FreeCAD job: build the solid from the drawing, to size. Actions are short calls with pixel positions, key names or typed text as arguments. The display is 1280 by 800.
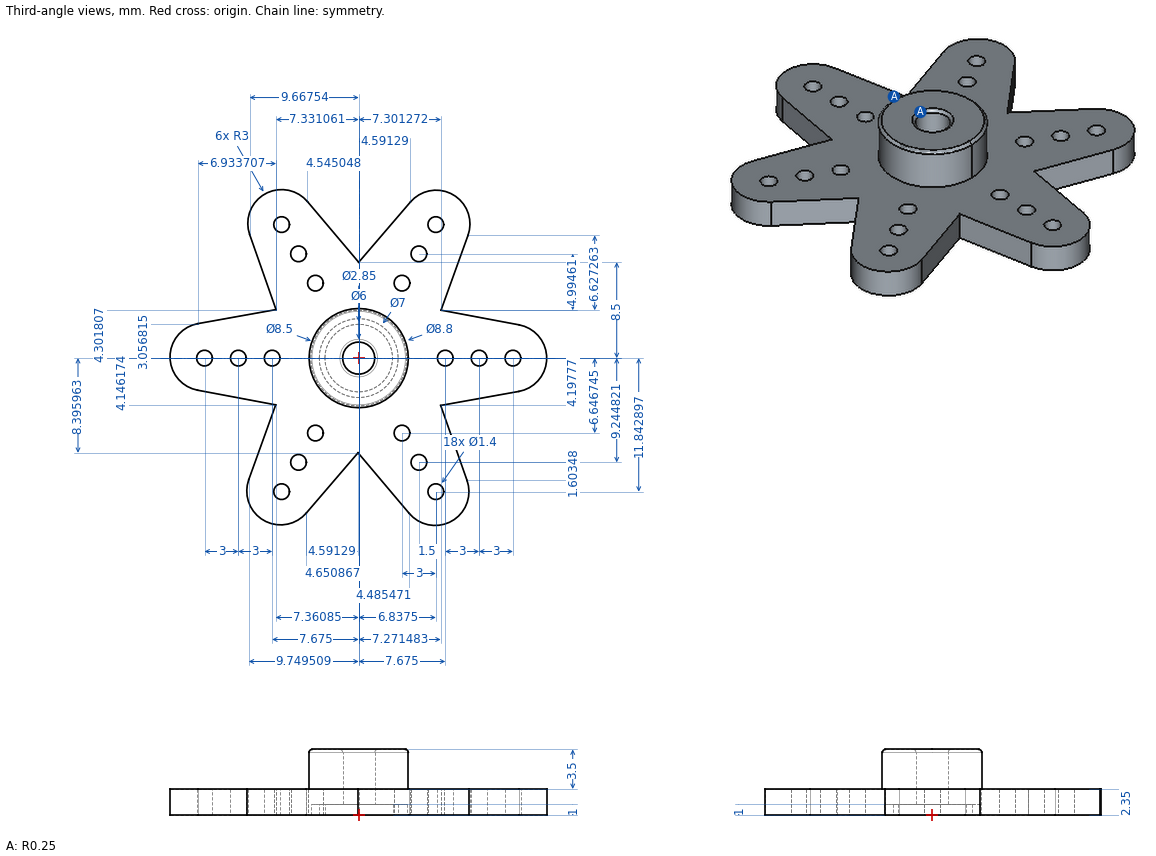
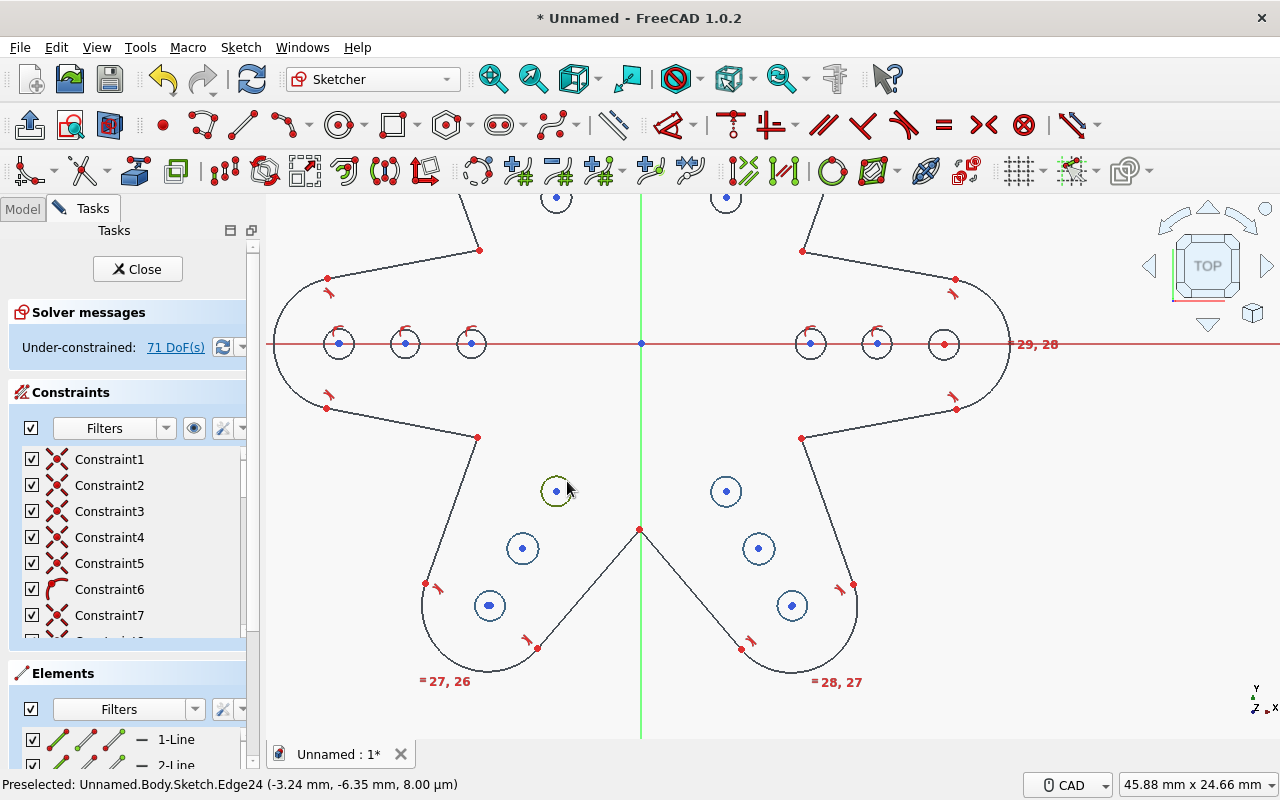
scroll(955, 334, up, 2)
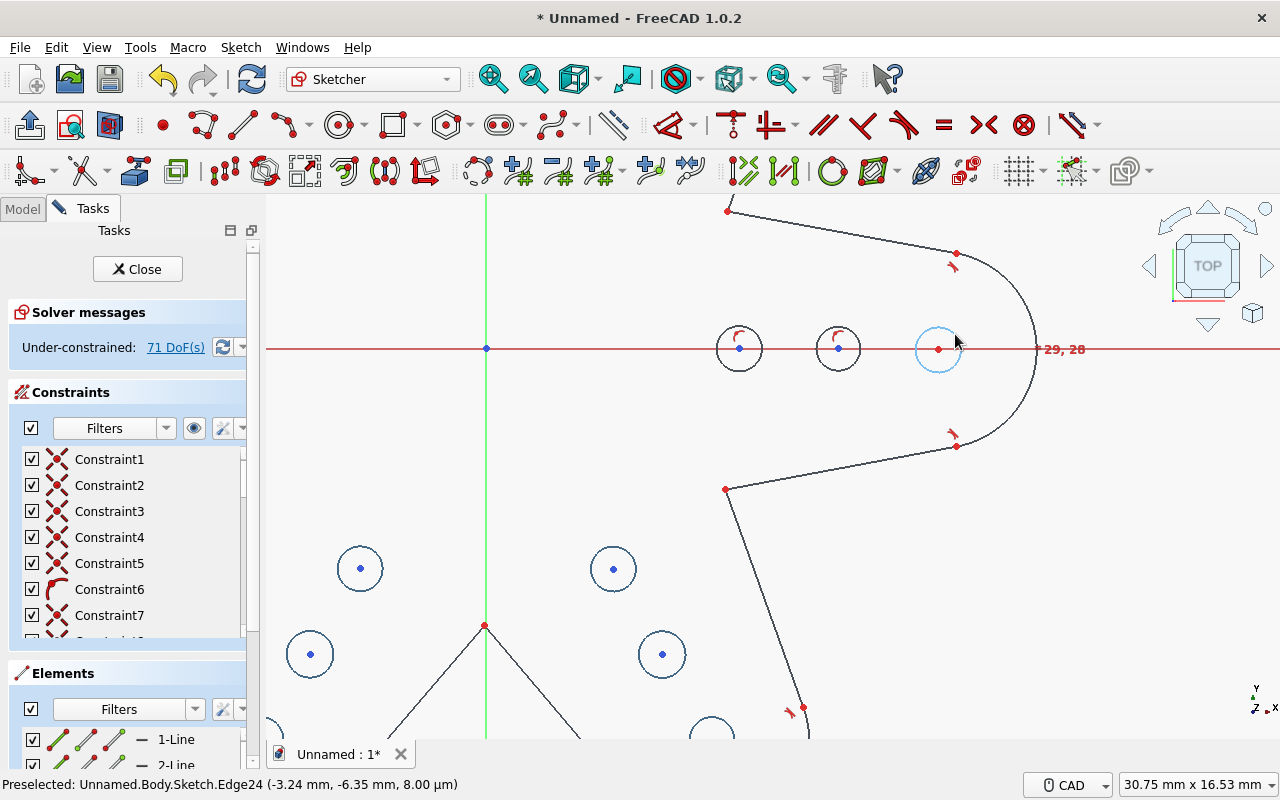
click(954, 334)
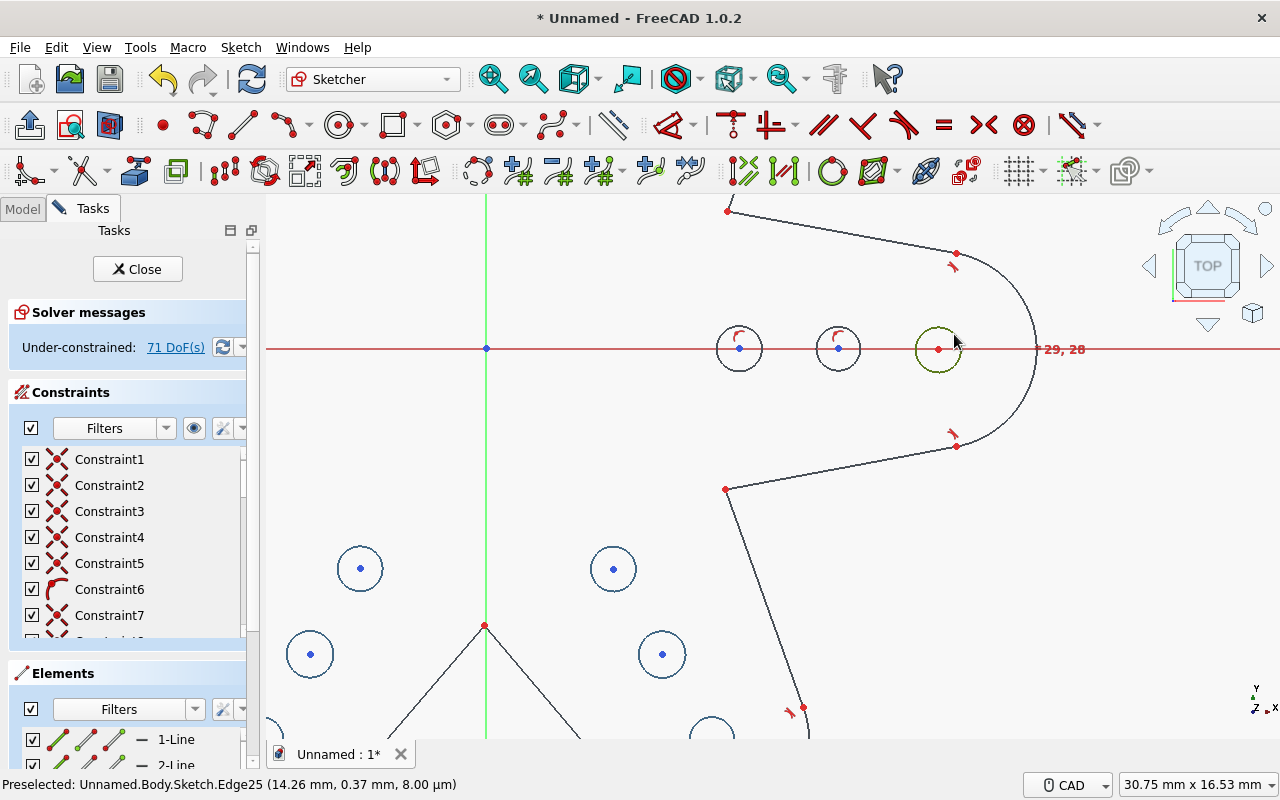
click(854, 333)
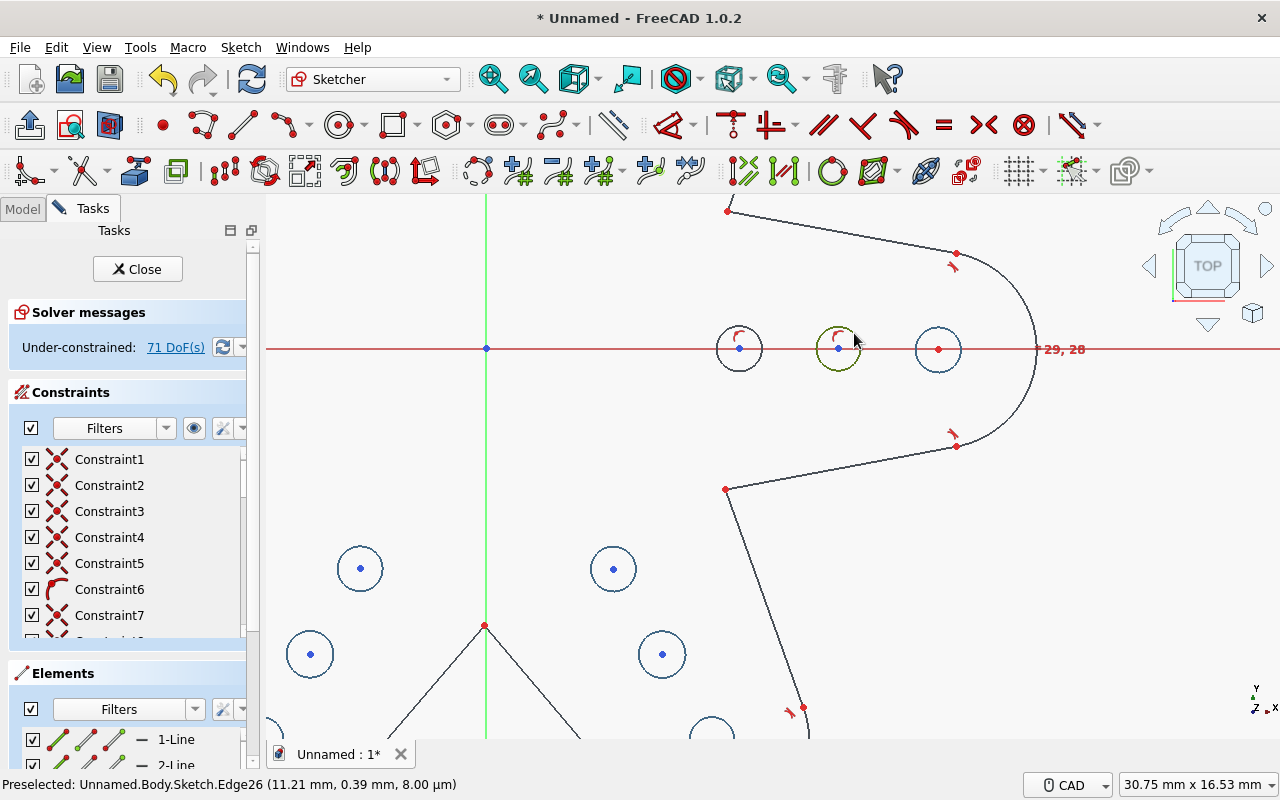
click(755, 333)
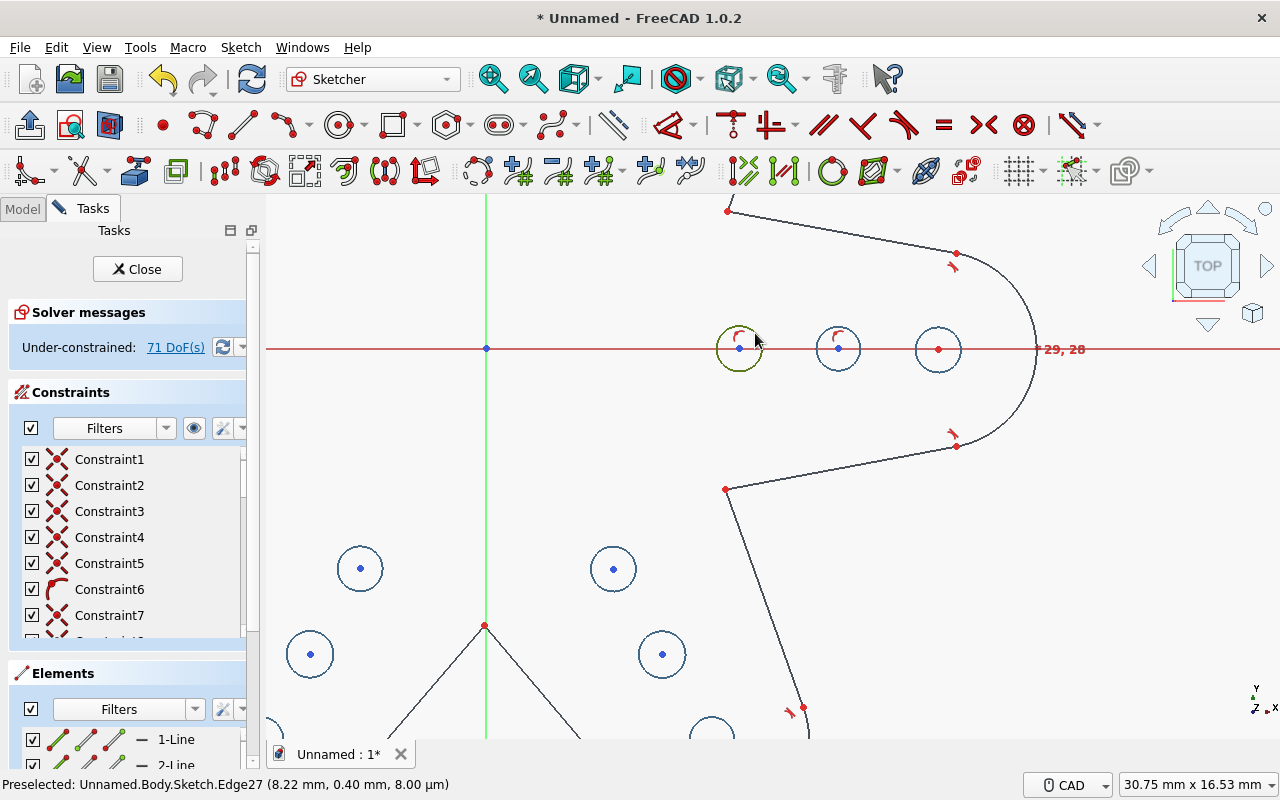
scroll(832, 536, down, 5)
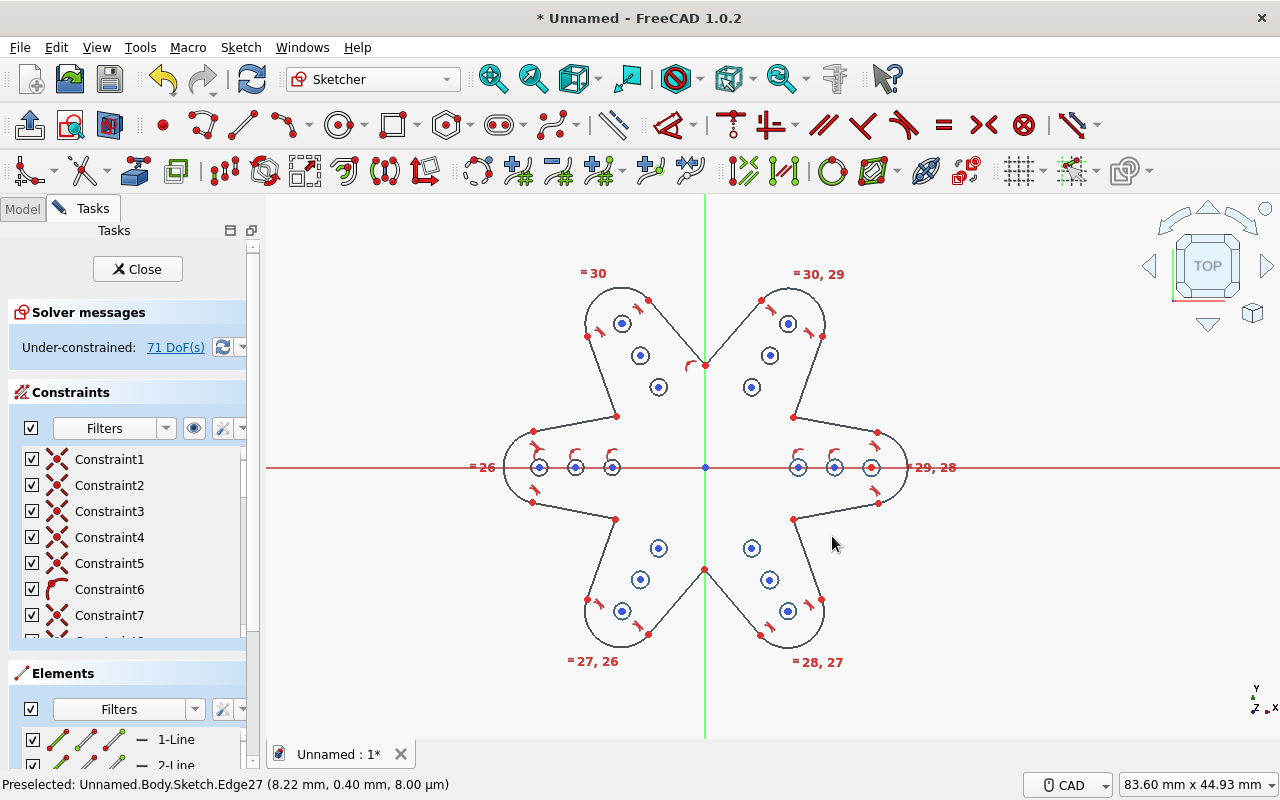
scroll(758, 381, up, 3)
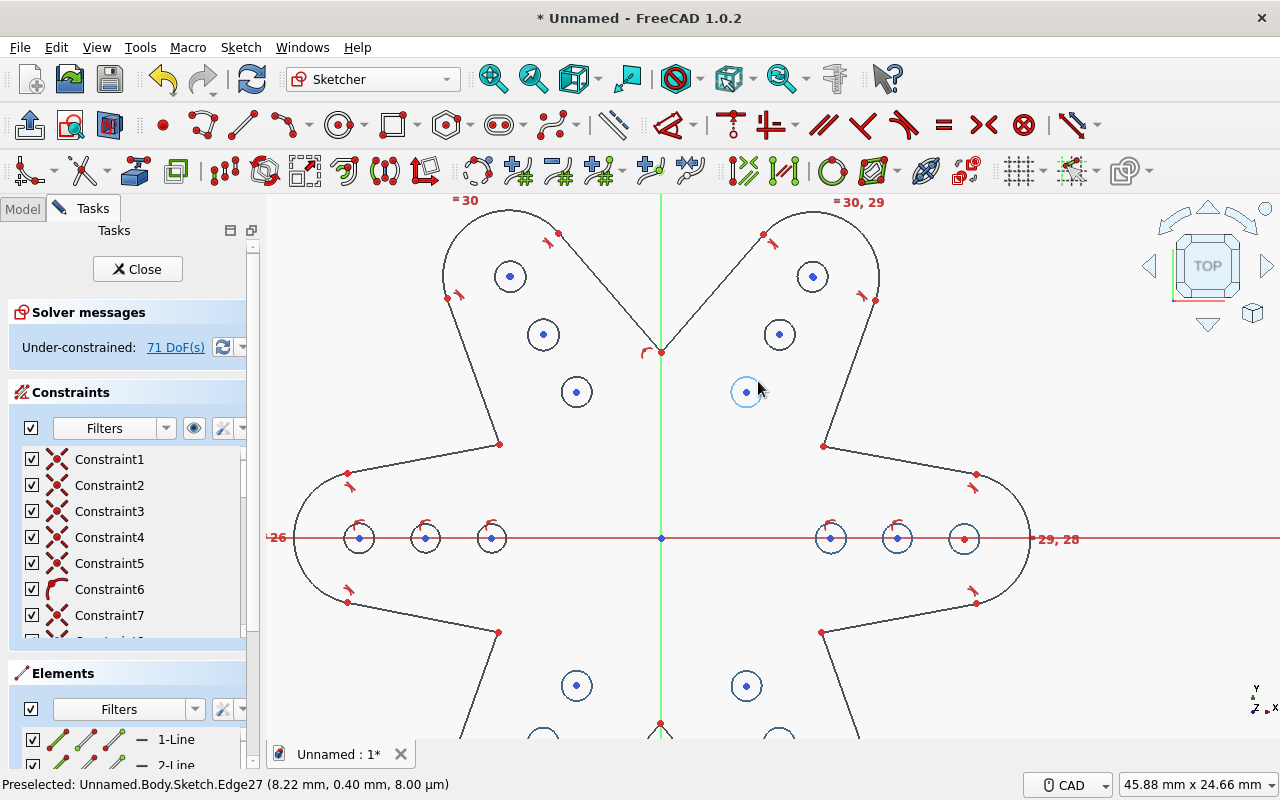
click(757, 381)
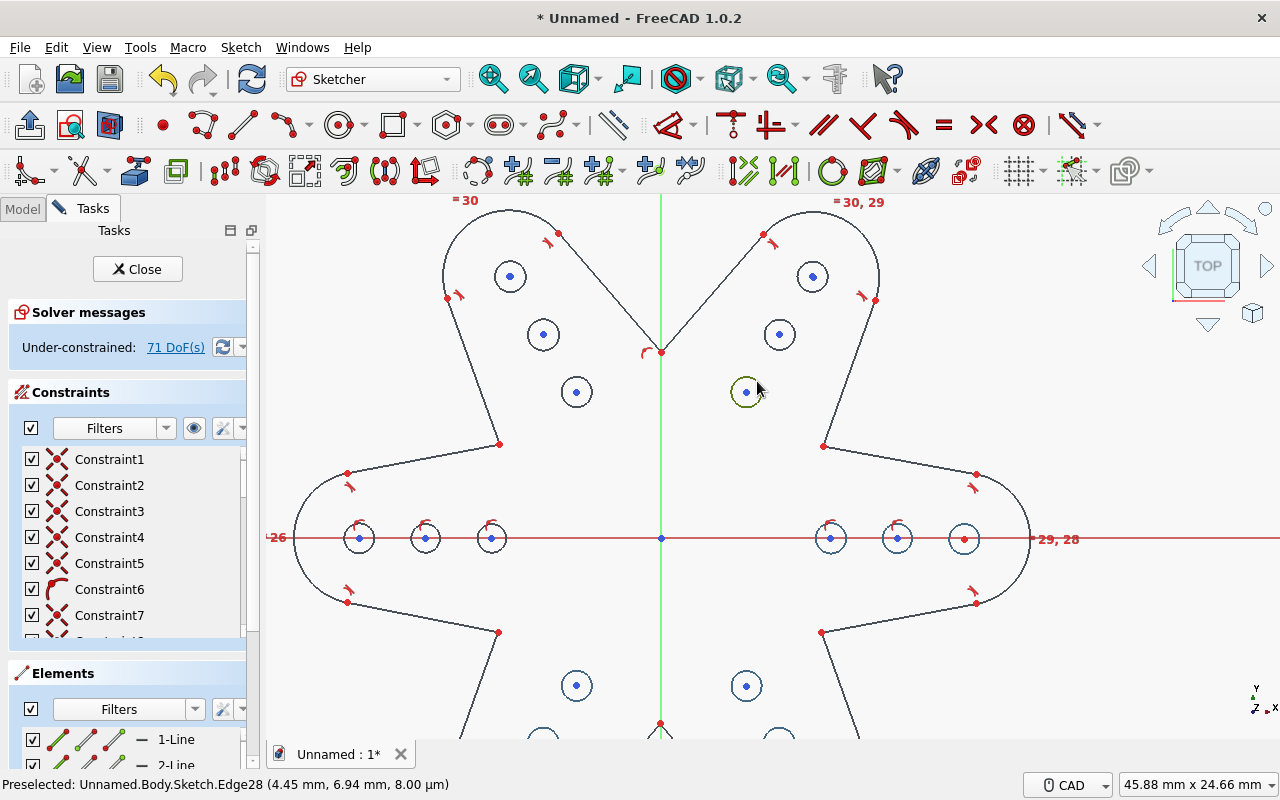
click(790, 324)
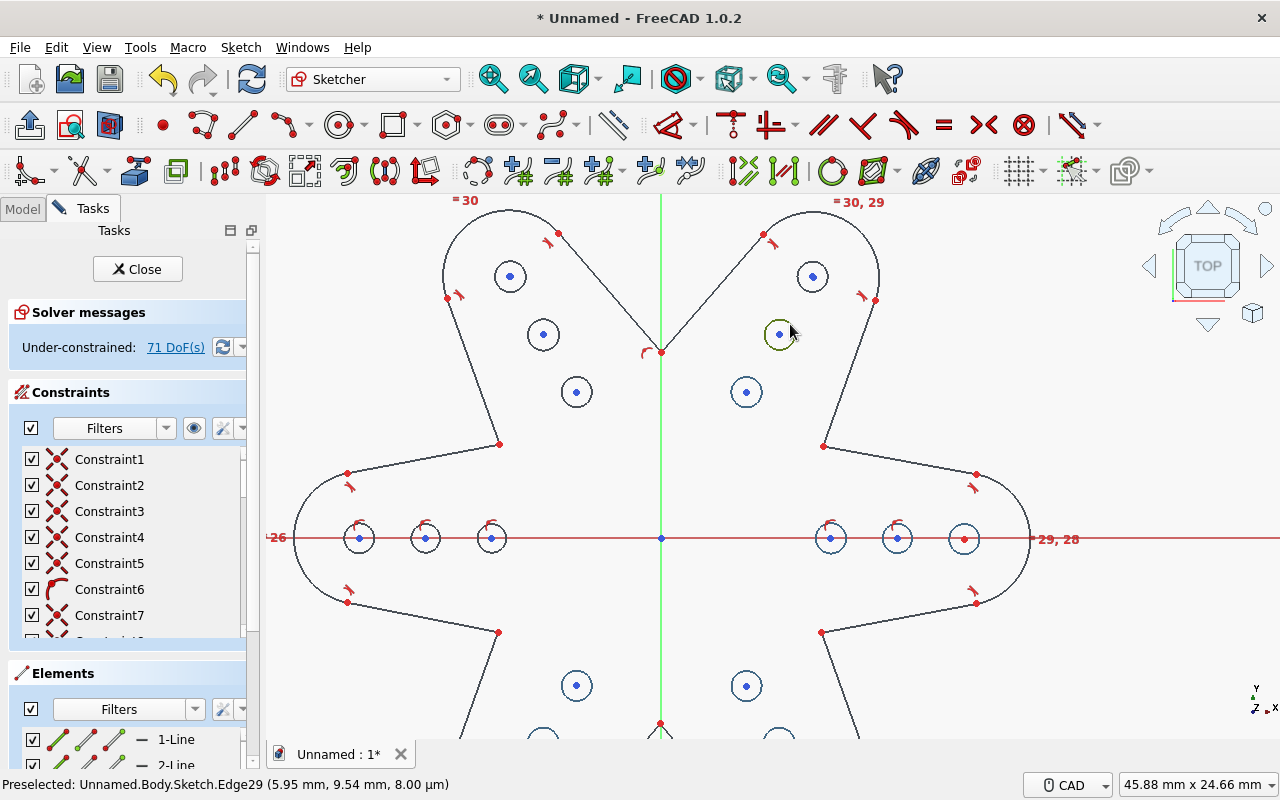
click(823, 266)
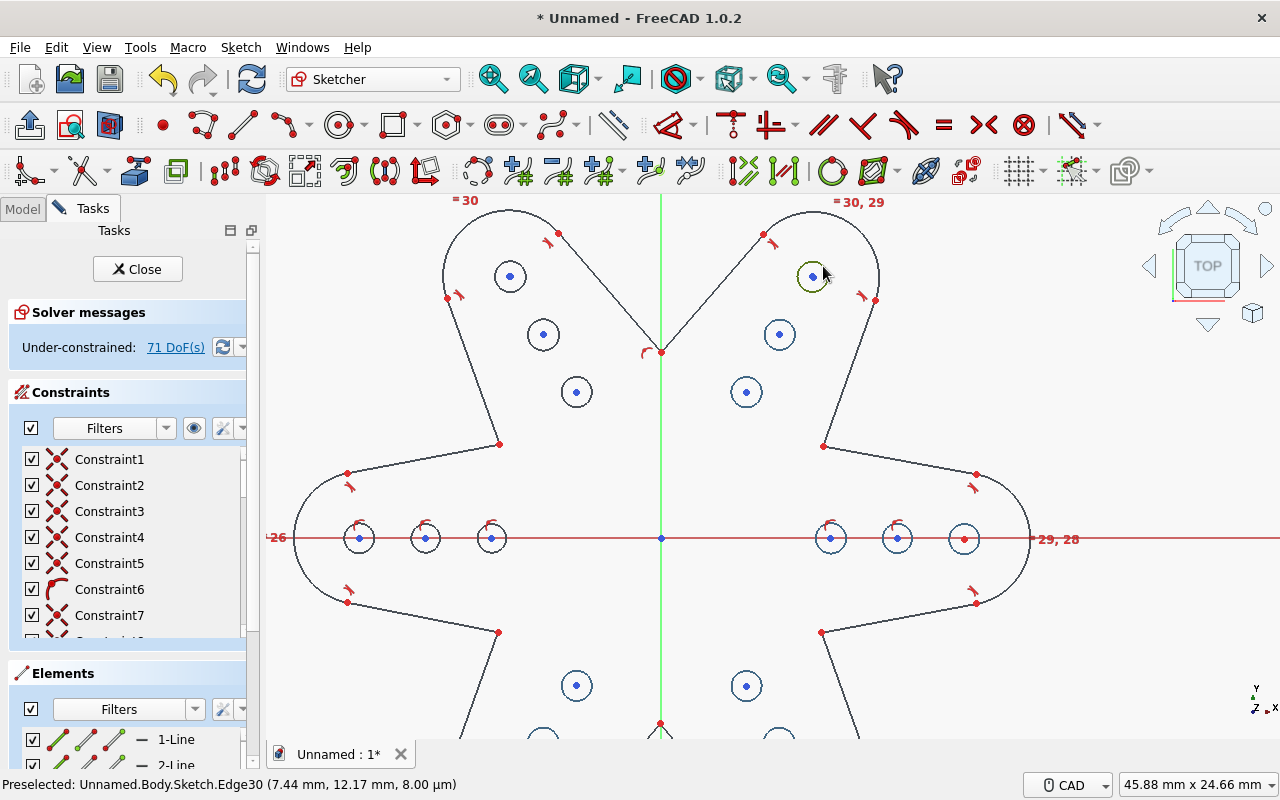
scroll(502, 528, up, 2)